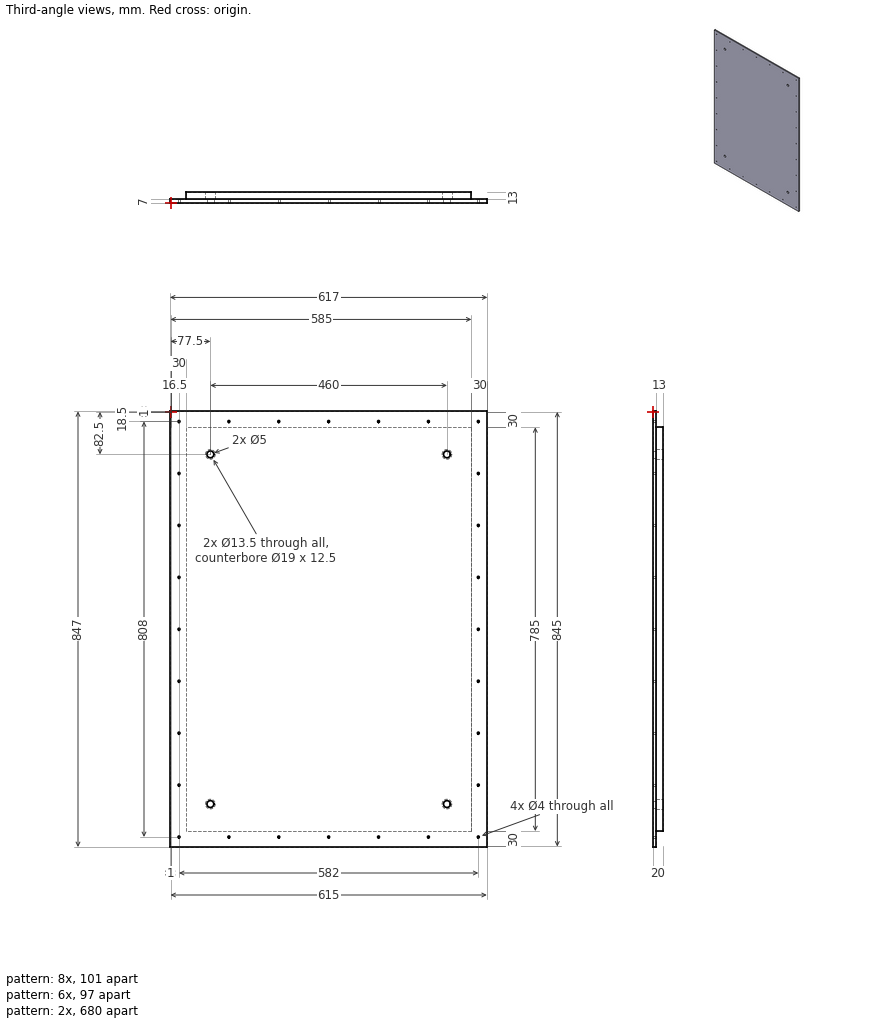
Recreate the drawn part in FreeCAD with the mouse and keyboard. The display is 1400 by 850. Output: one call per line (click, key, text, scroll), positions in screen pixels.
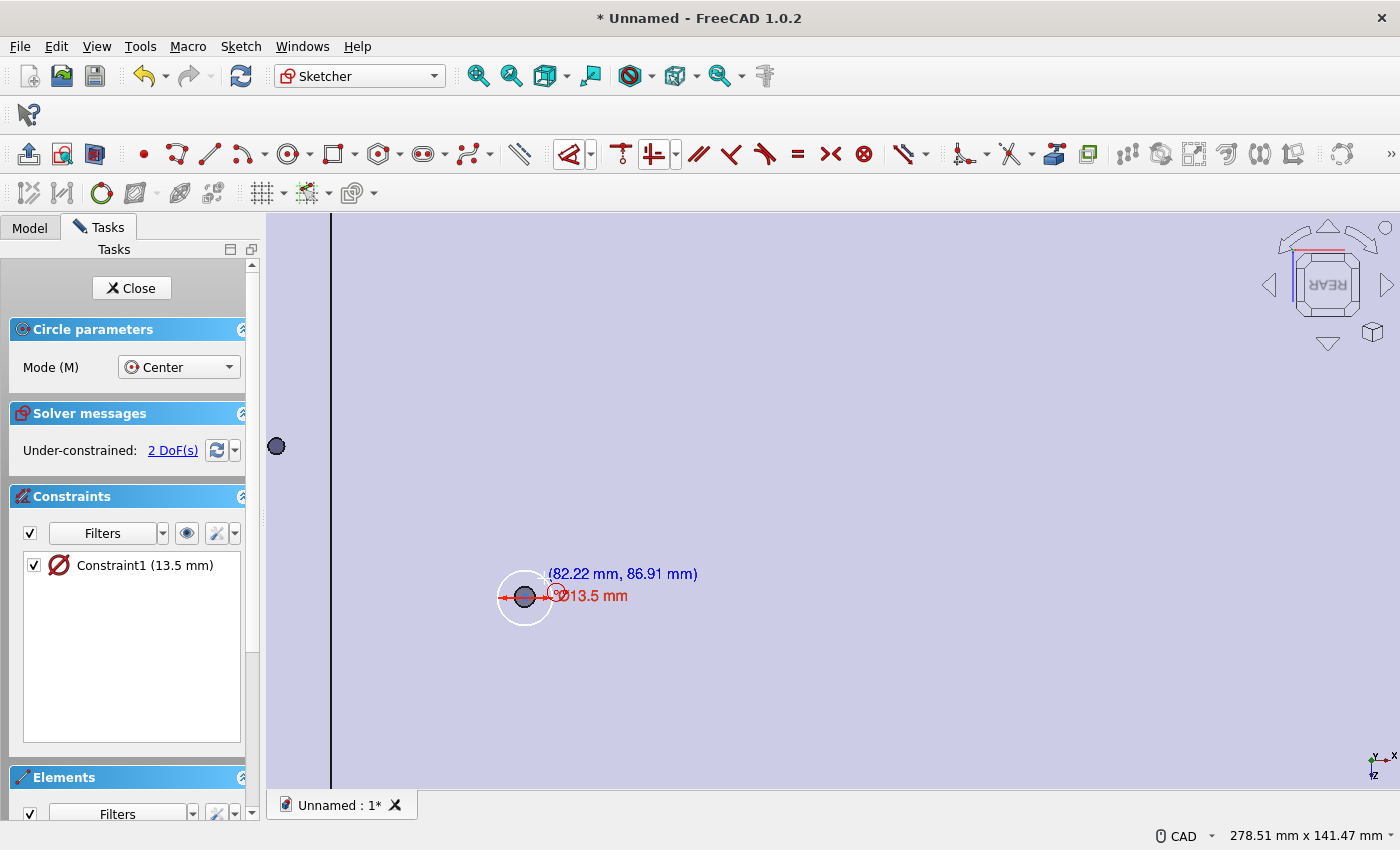
scroll(526, 393, down, 6)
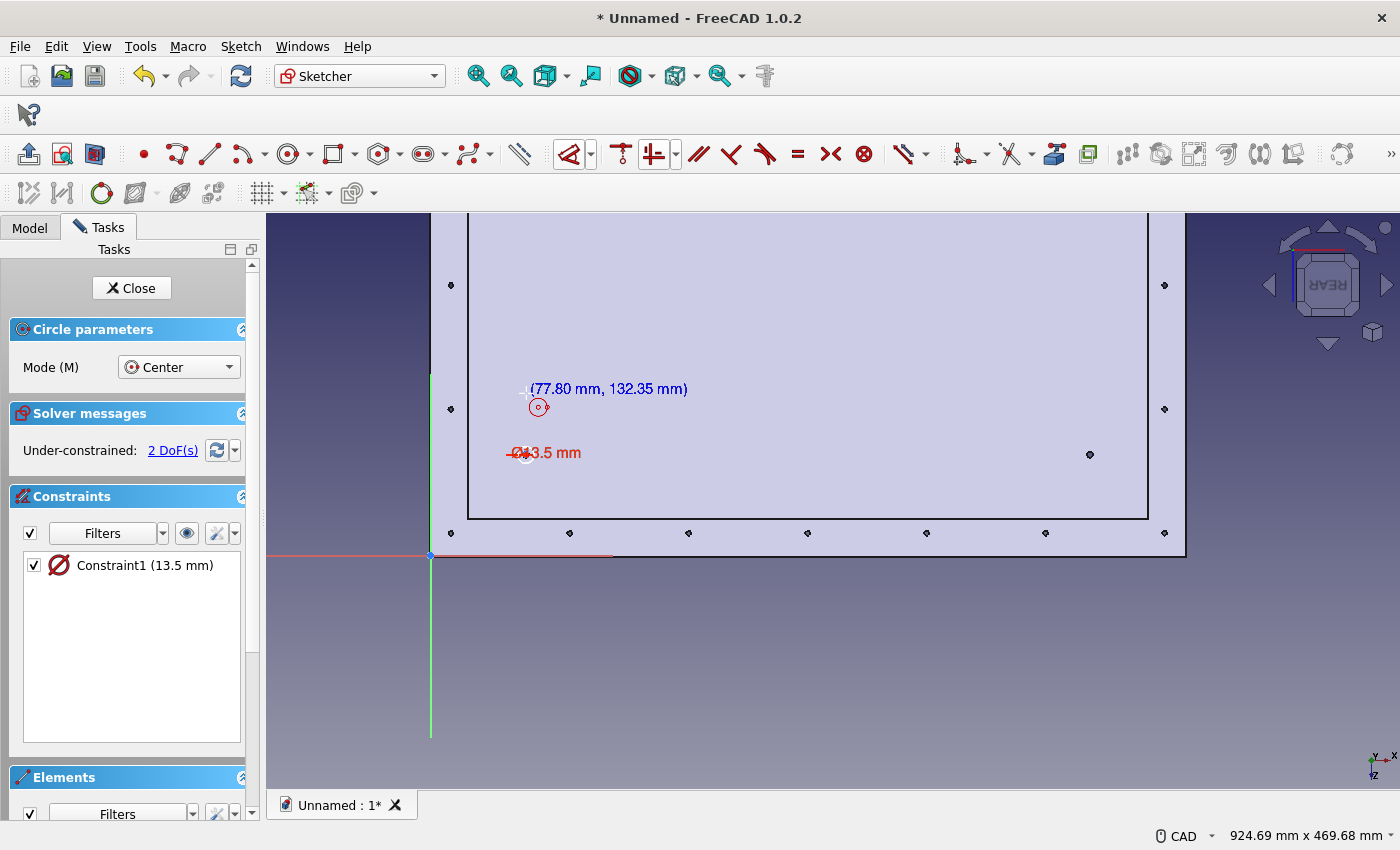
scroll(1090, 455, up, 6)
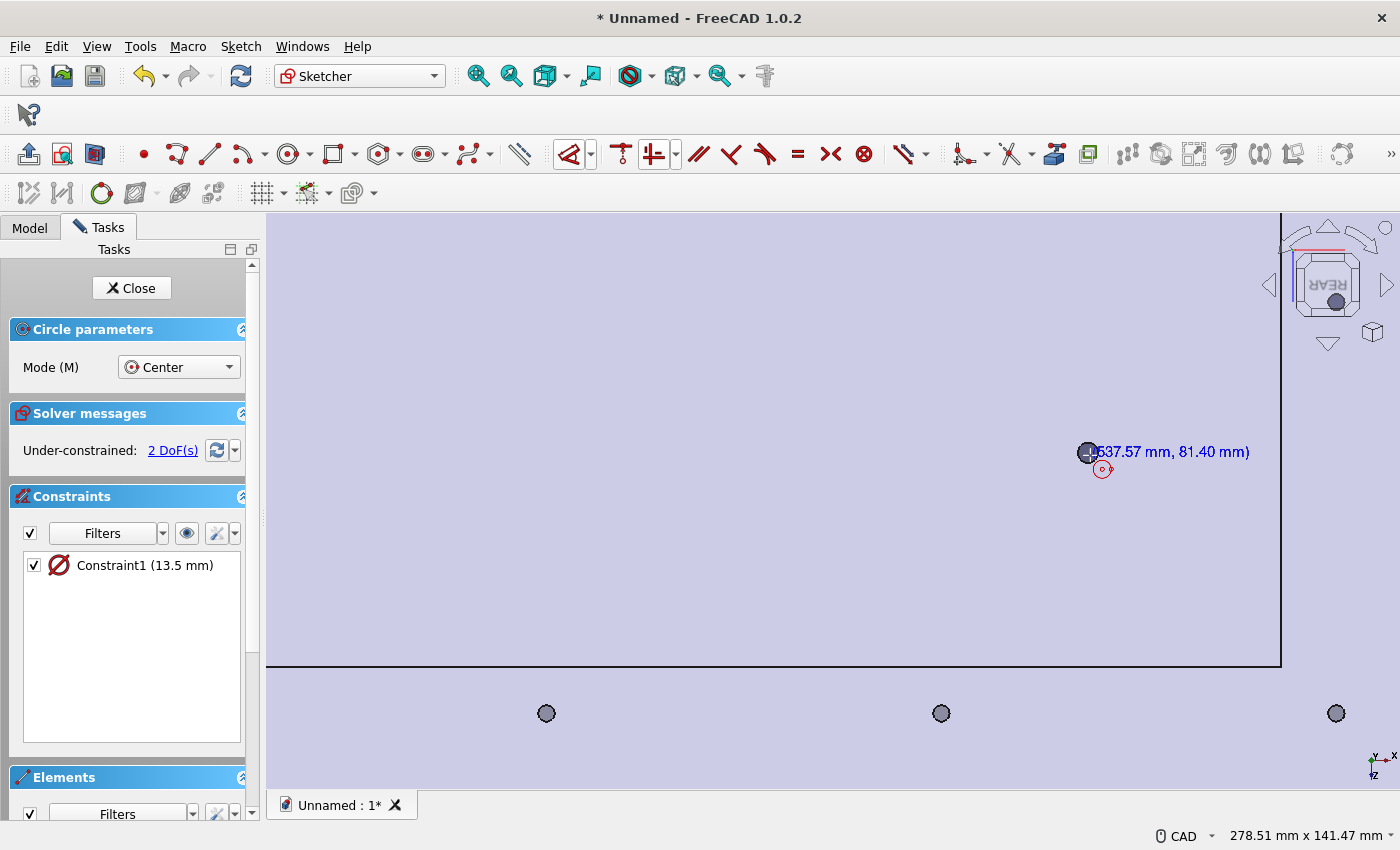
click(1088, 453)
move(1107, 433)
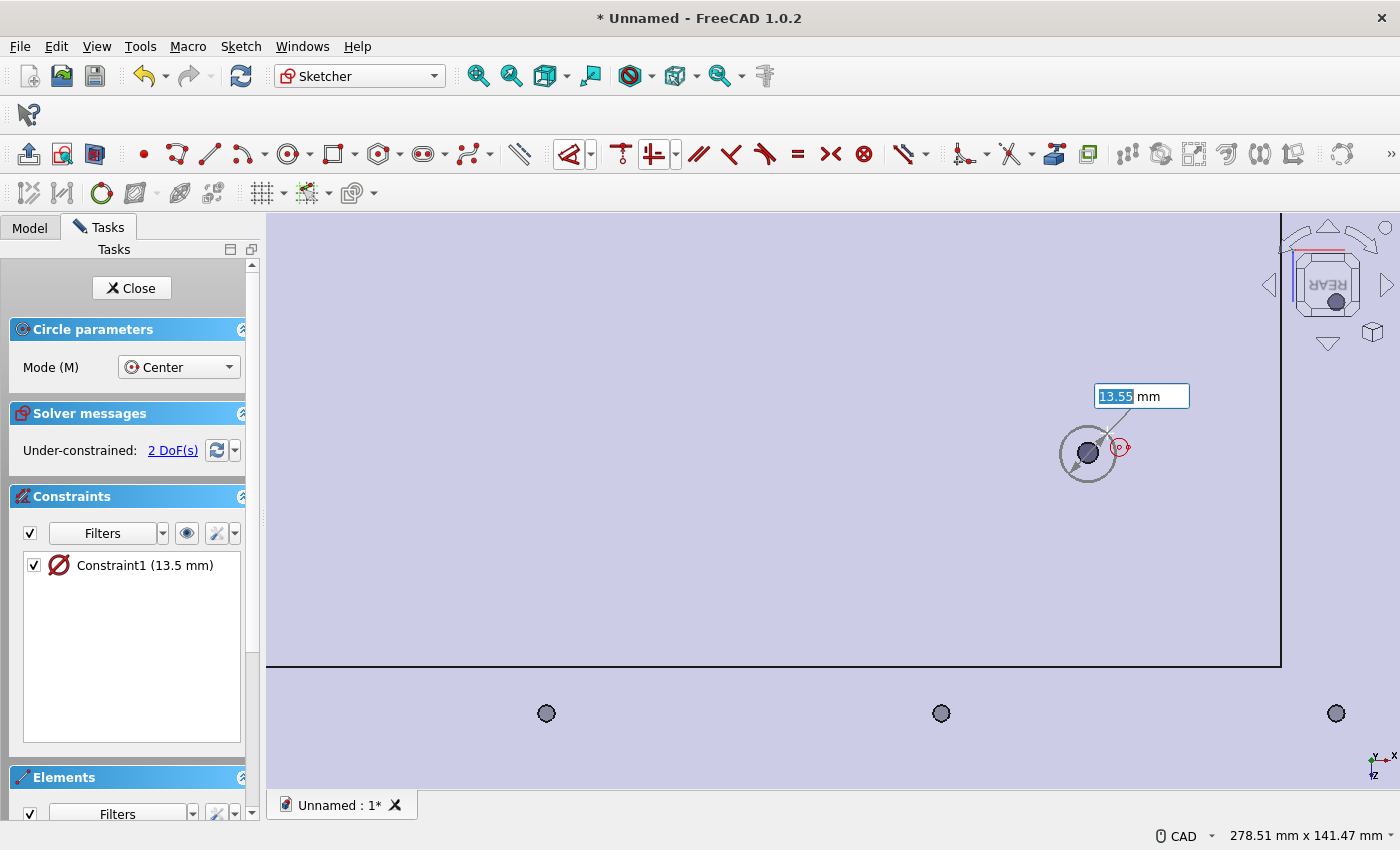
text(13.5)
key(Return)
key(Escape)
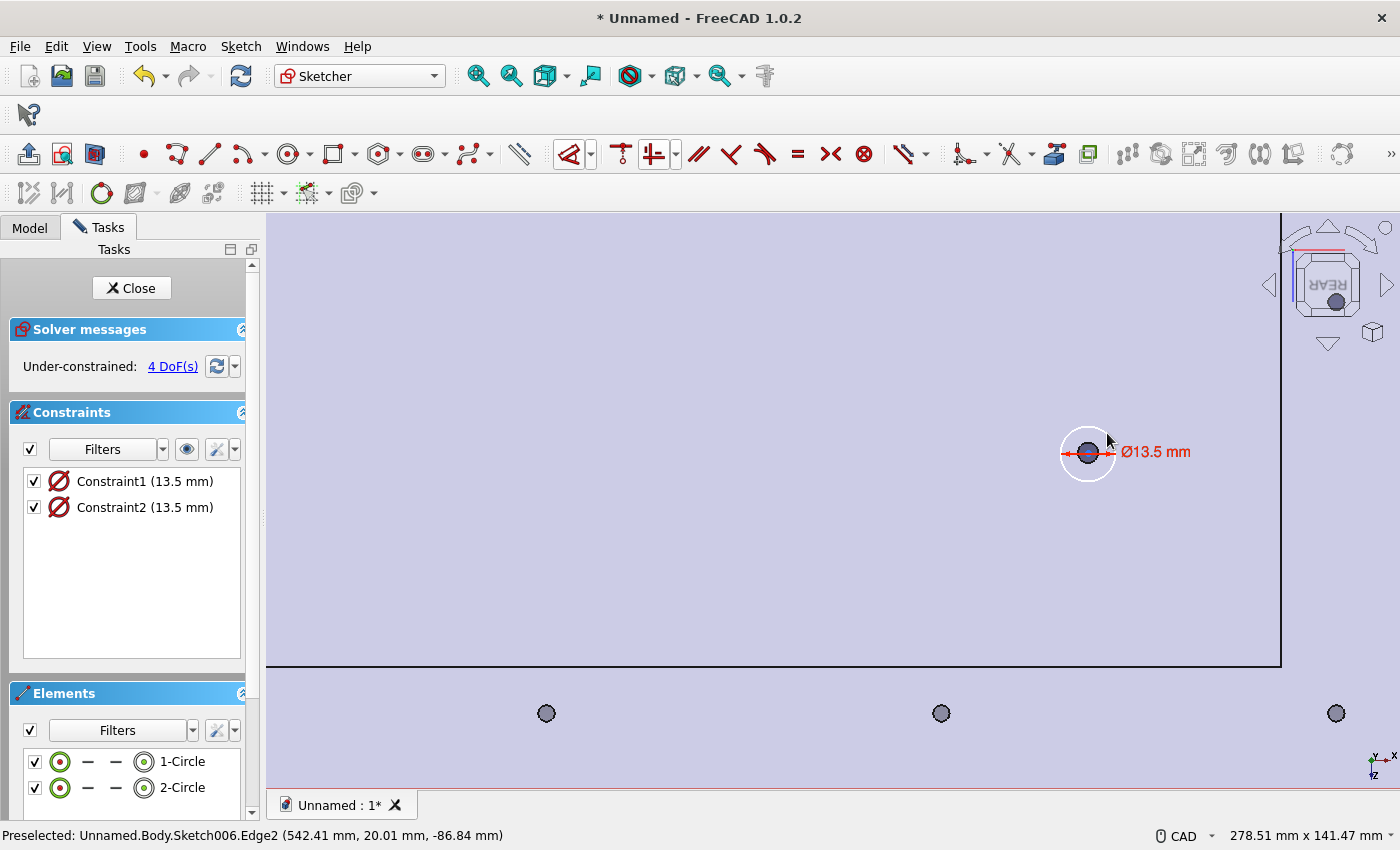
scroll(1091, 455, down, 6)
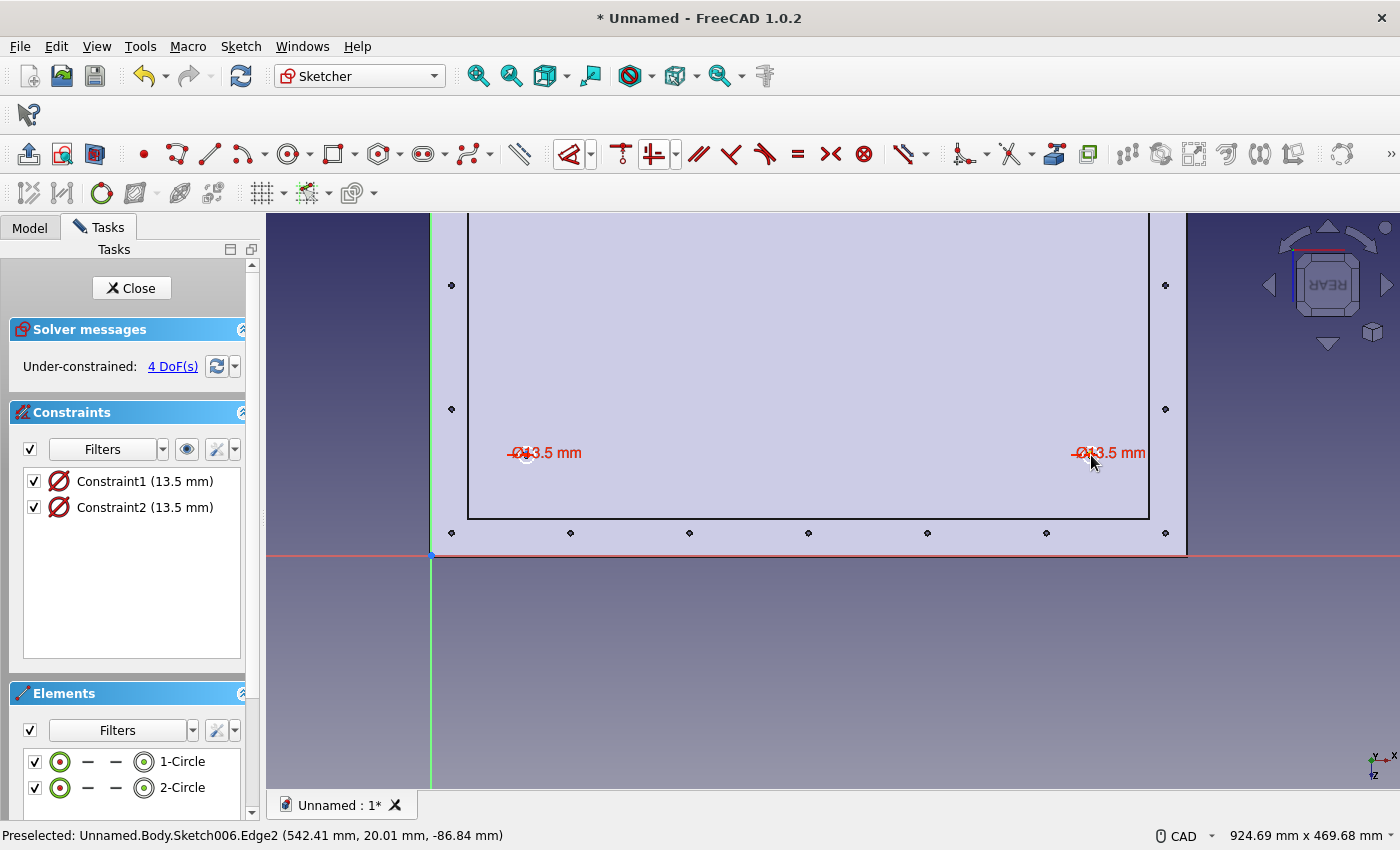
click(527, 455)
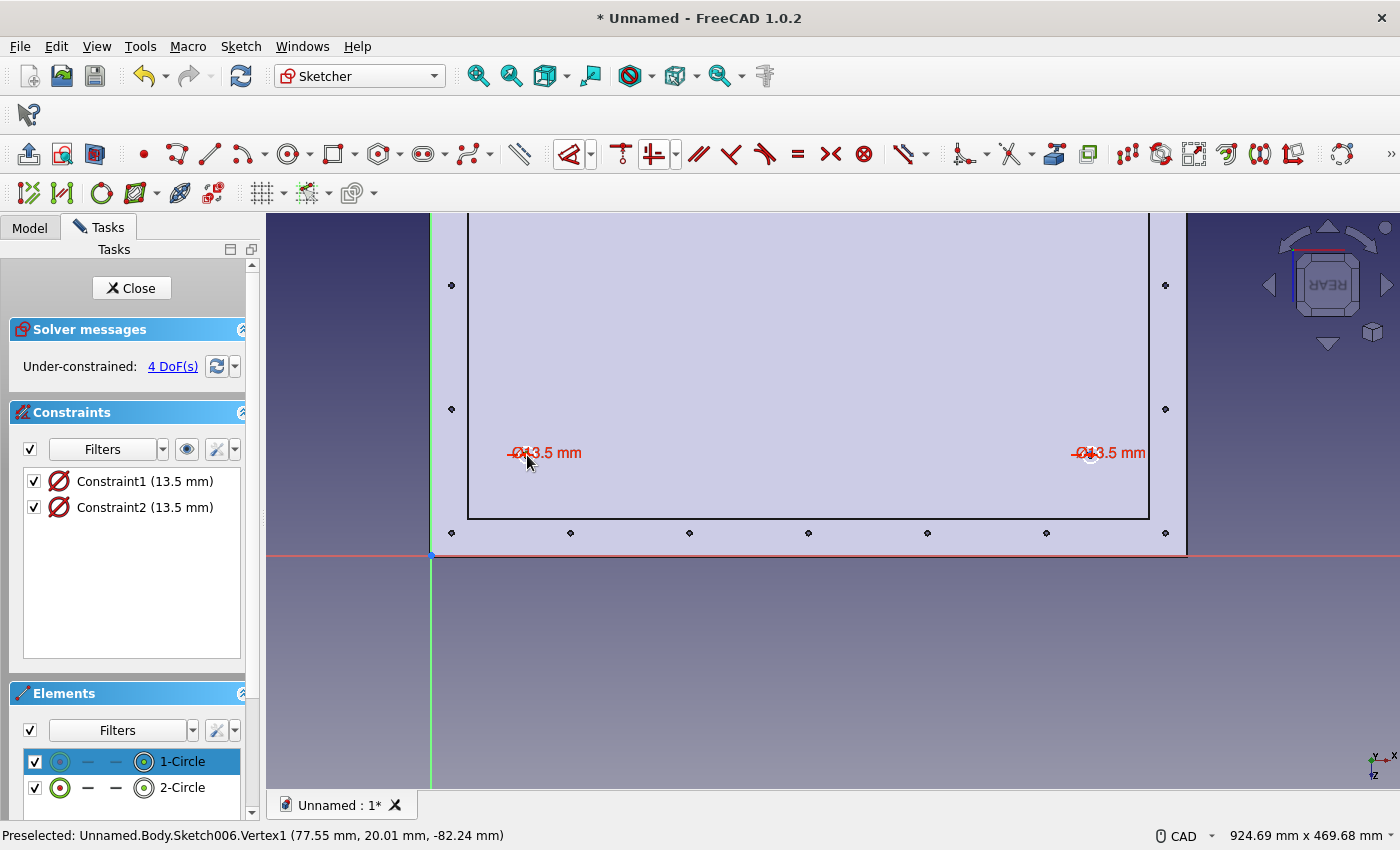
click(1091, 455)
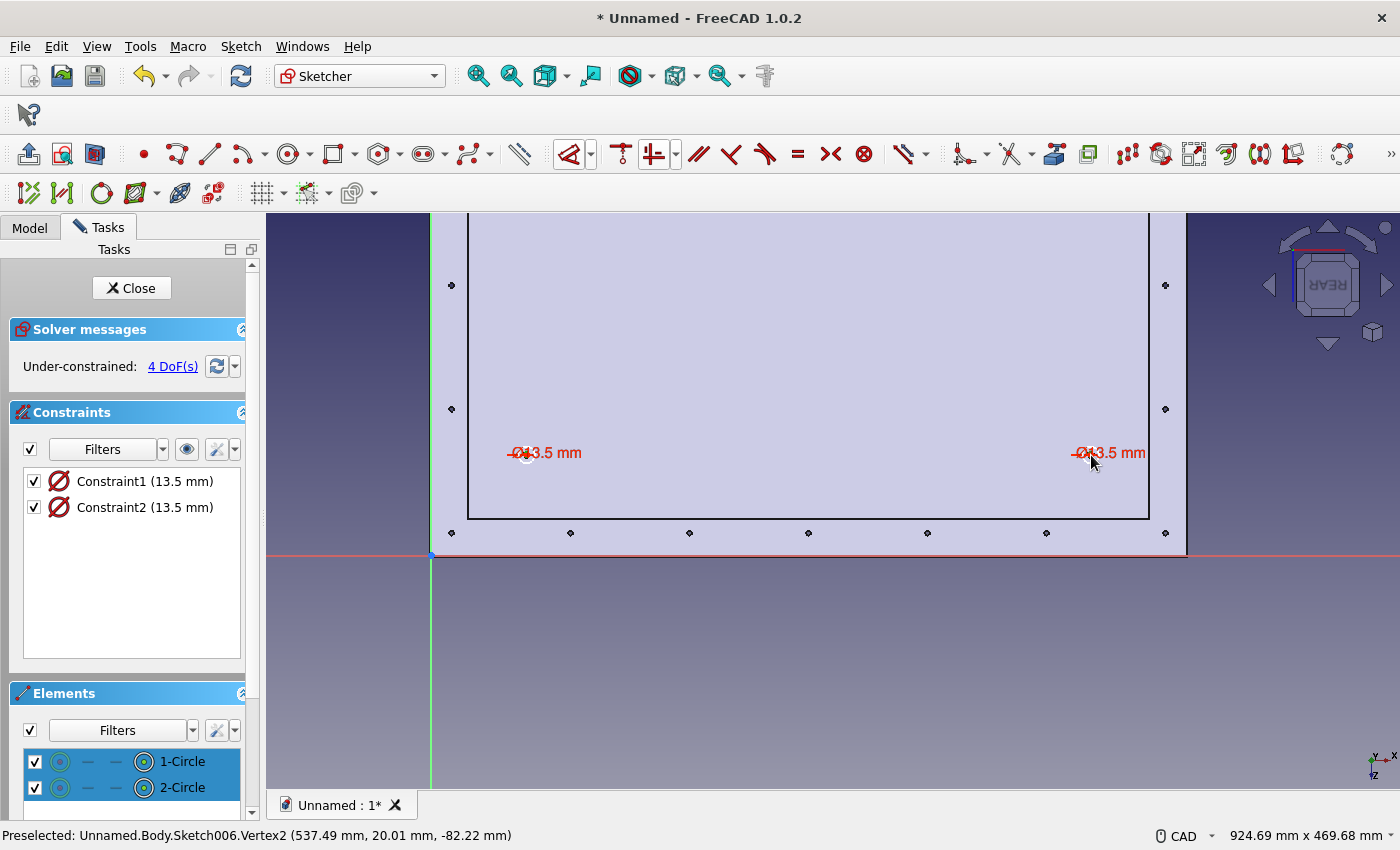
key(h)